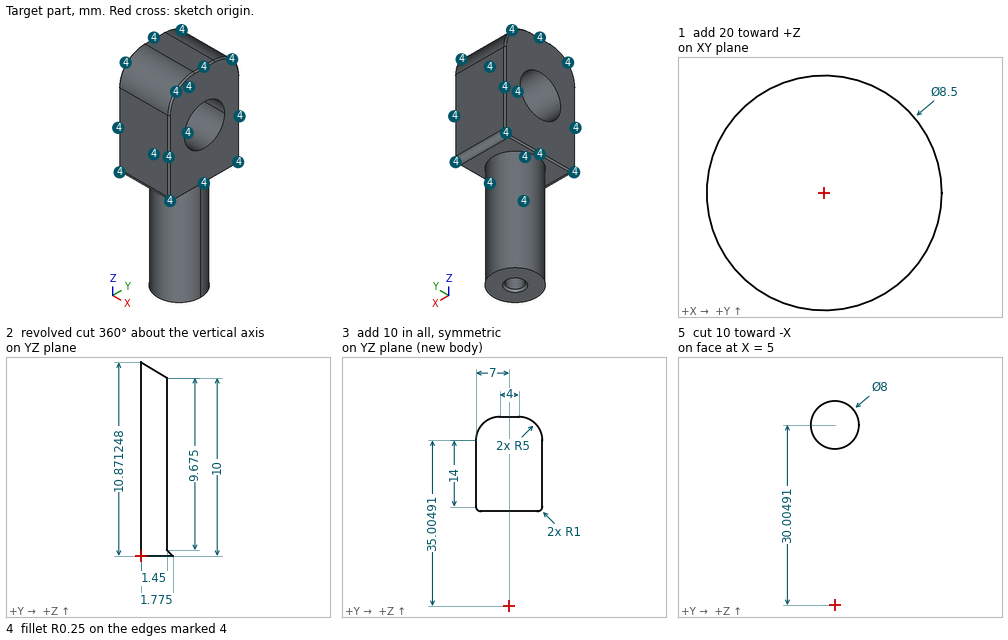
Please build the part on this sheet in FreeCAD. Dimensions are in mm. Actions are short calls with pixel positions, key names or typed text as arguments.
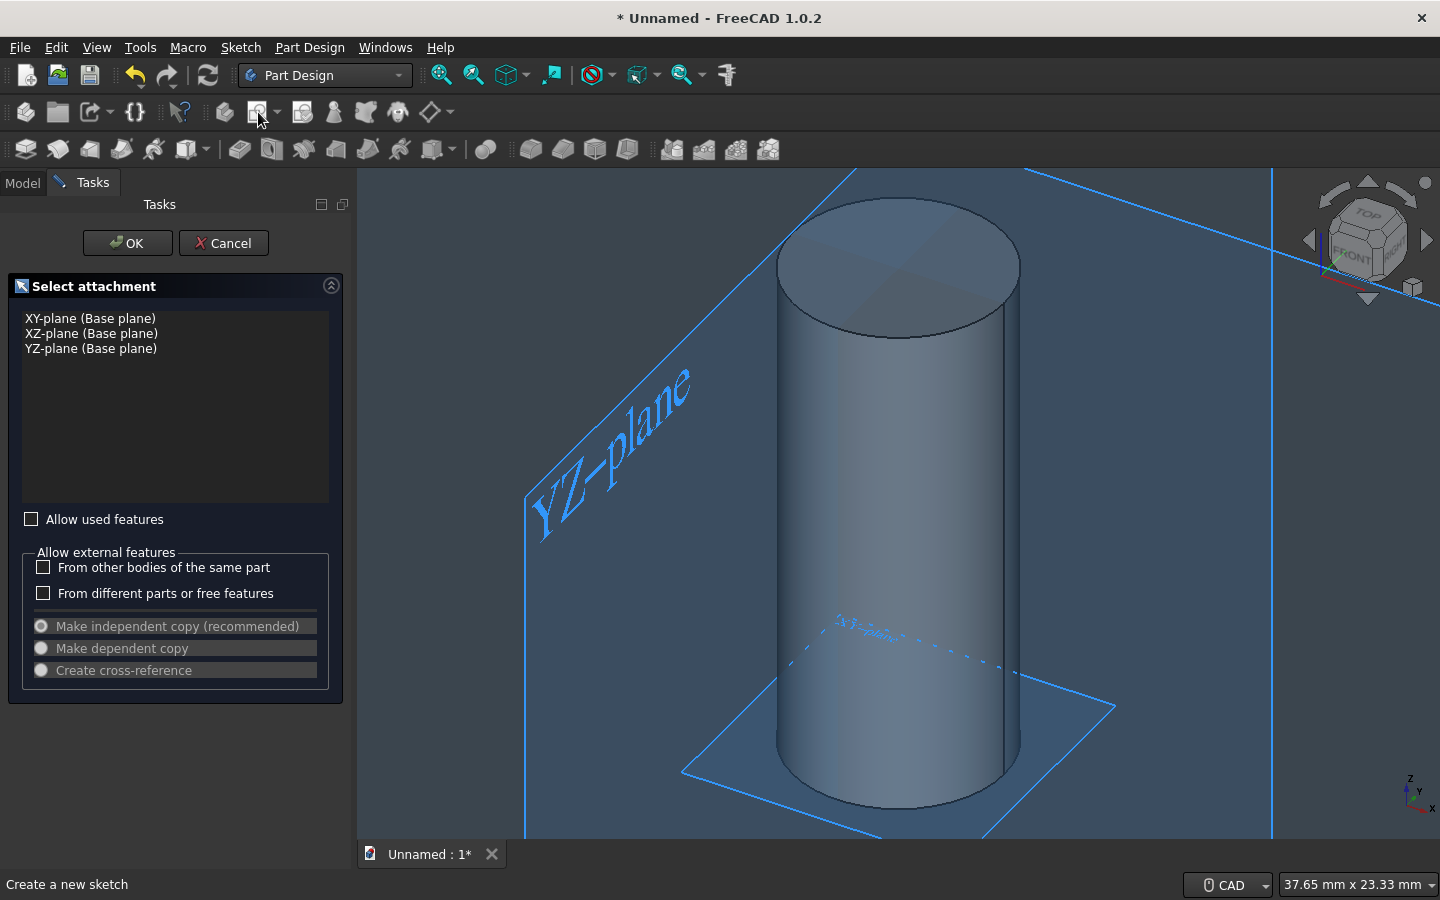
click(82, 348)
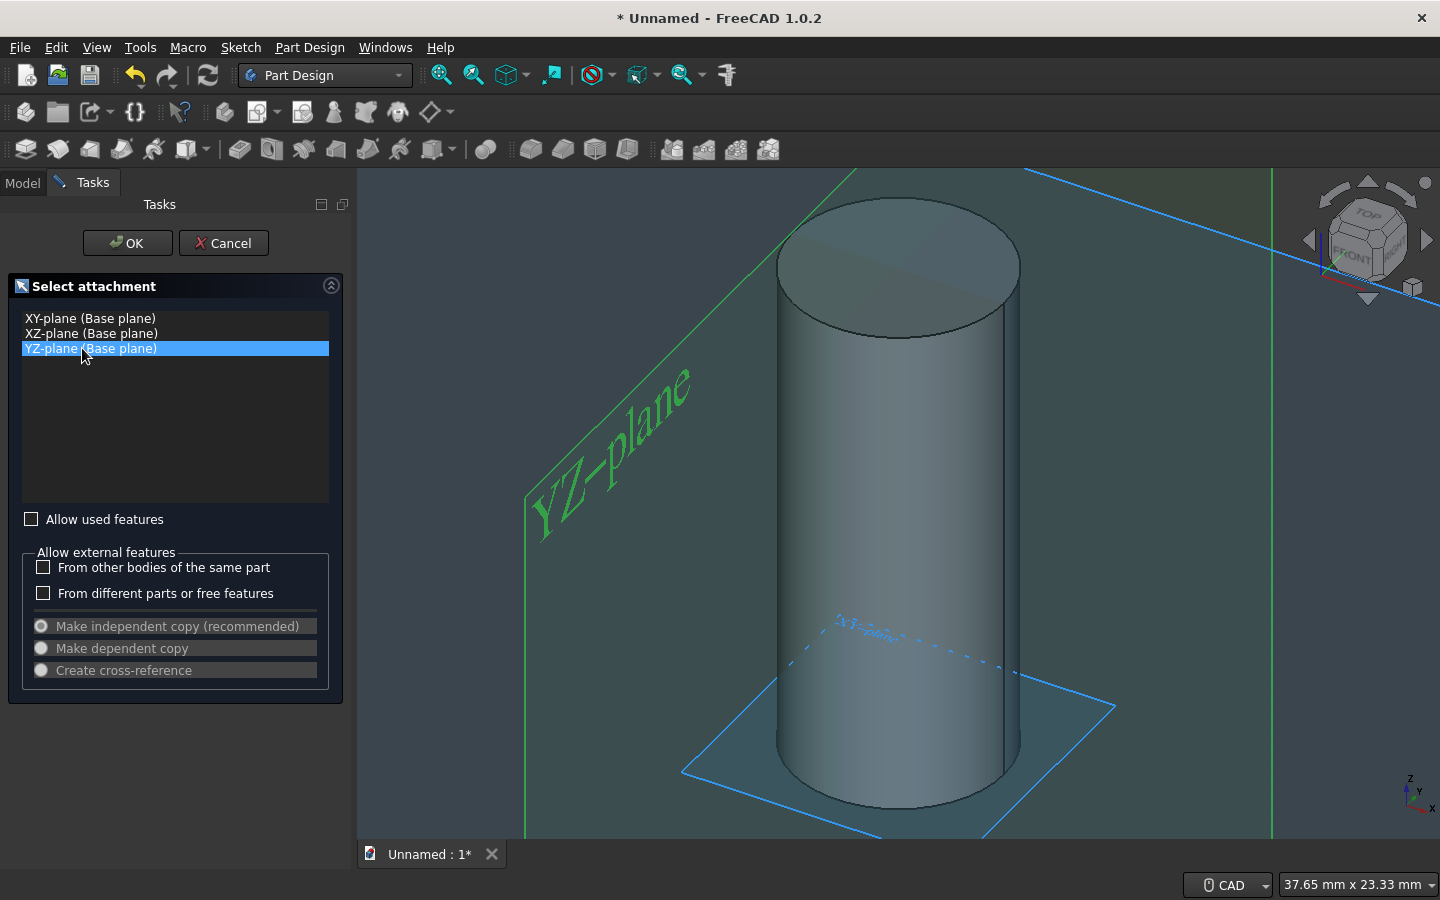
click(128, 243)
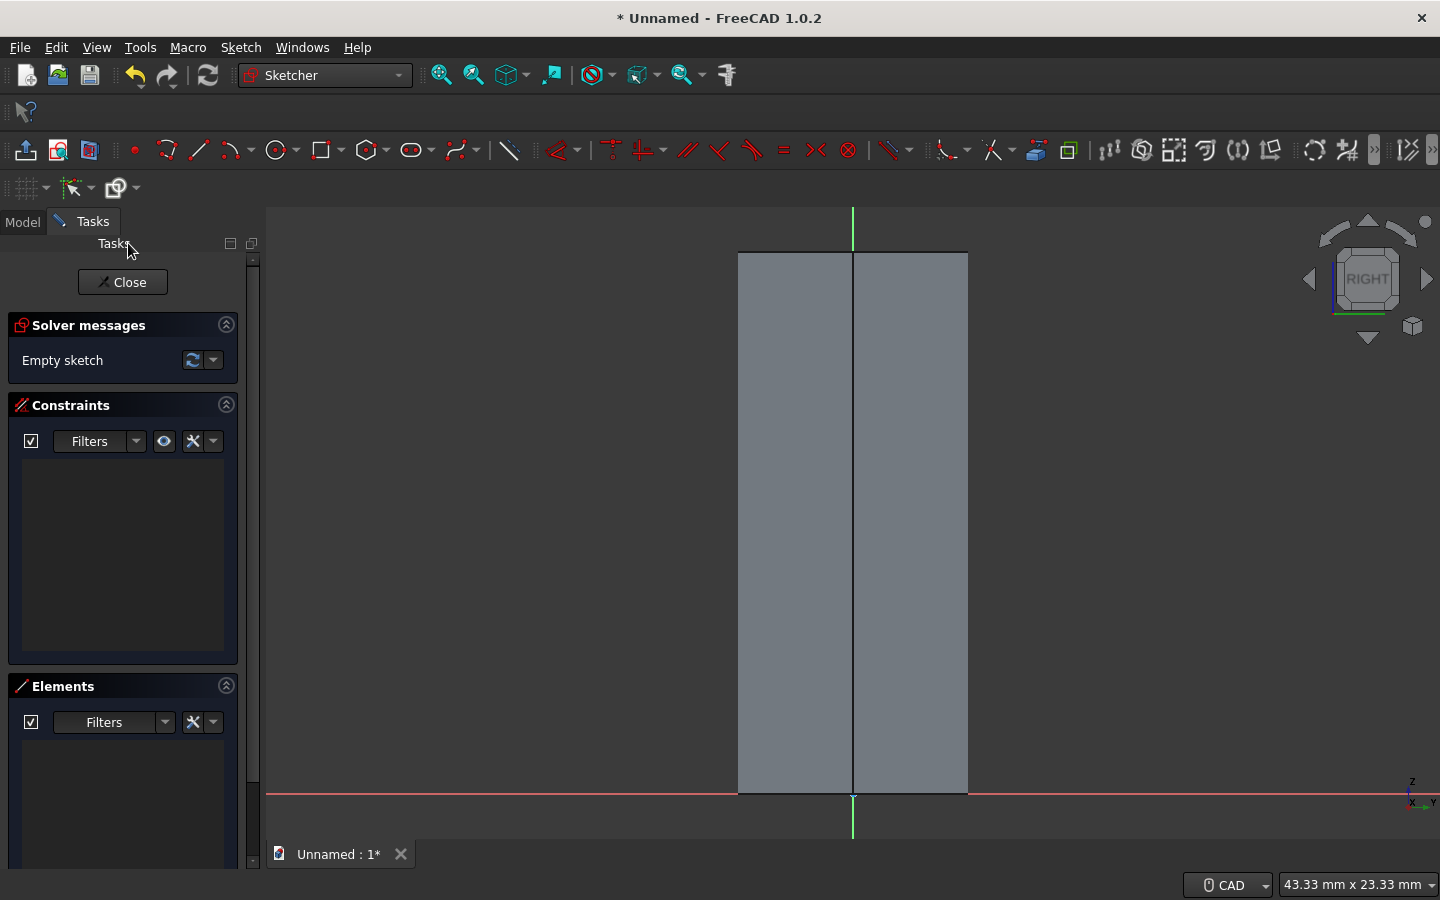
click(90, 150)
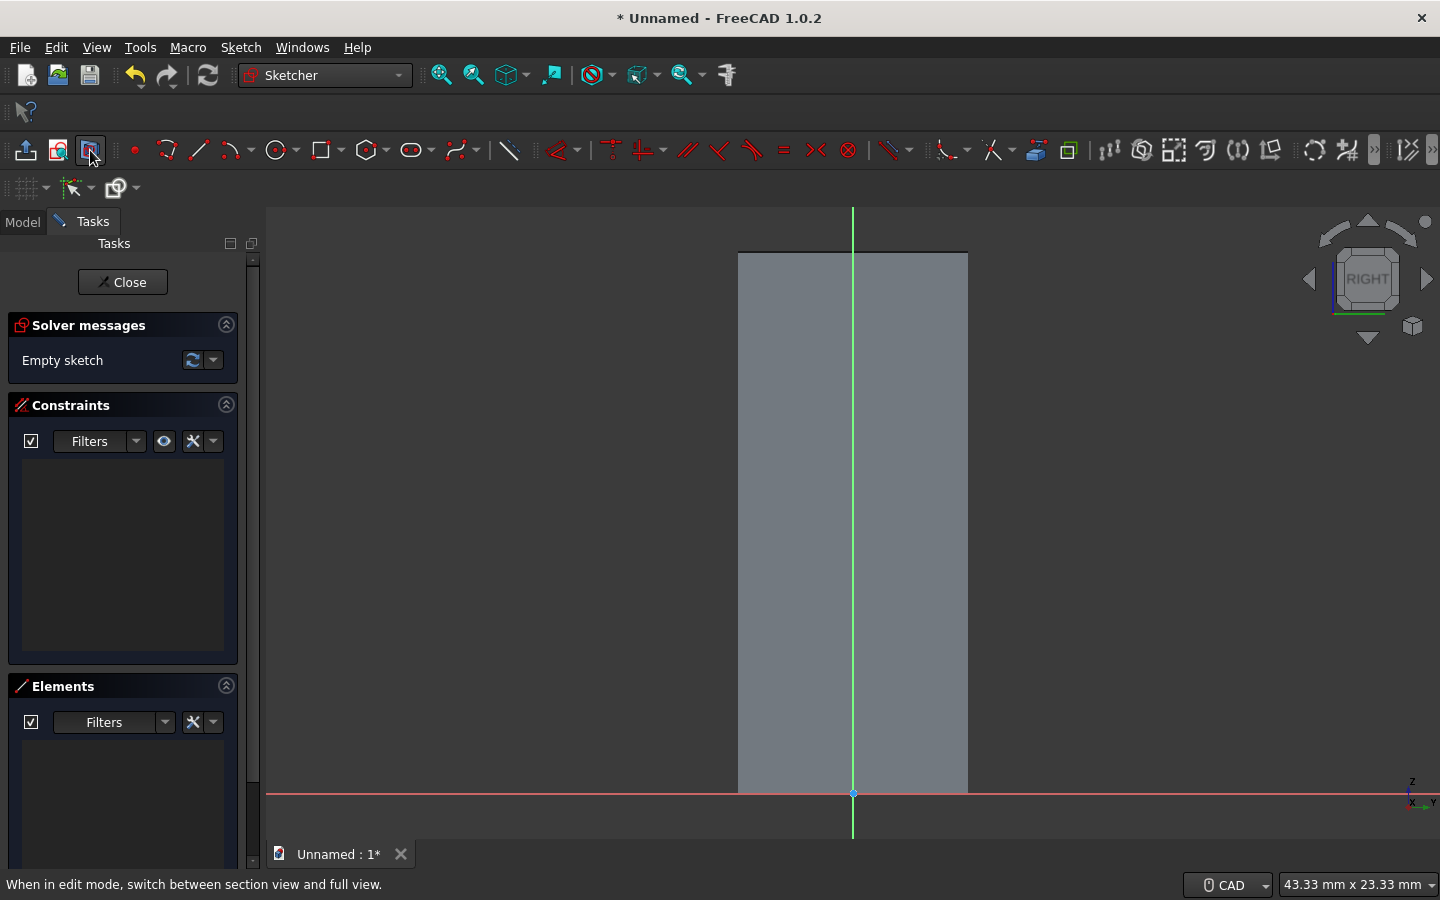
scroll(1065, 811, up, 2)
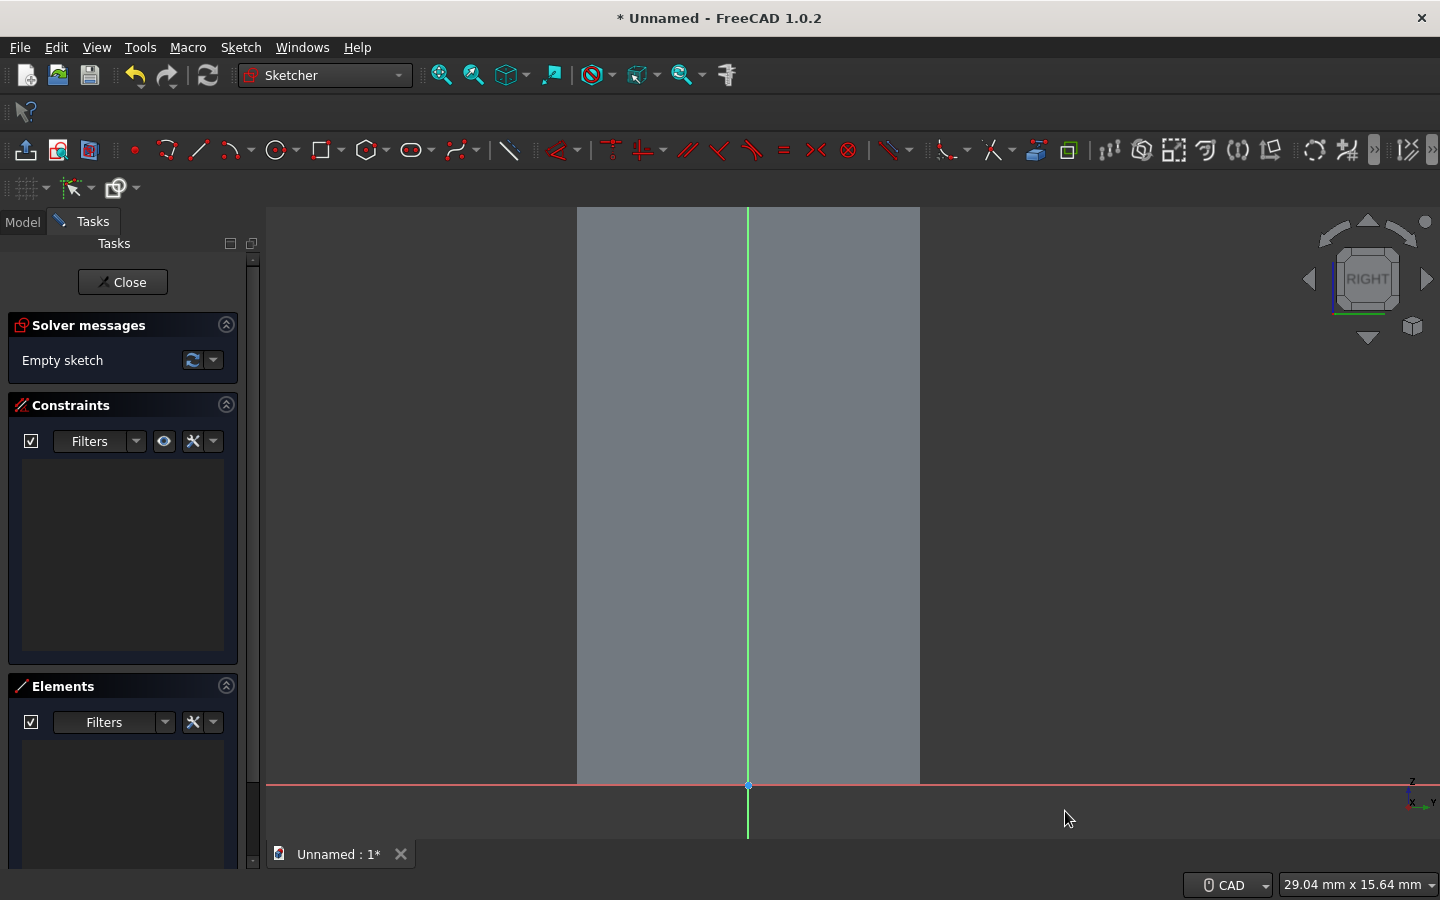
click(168, 150)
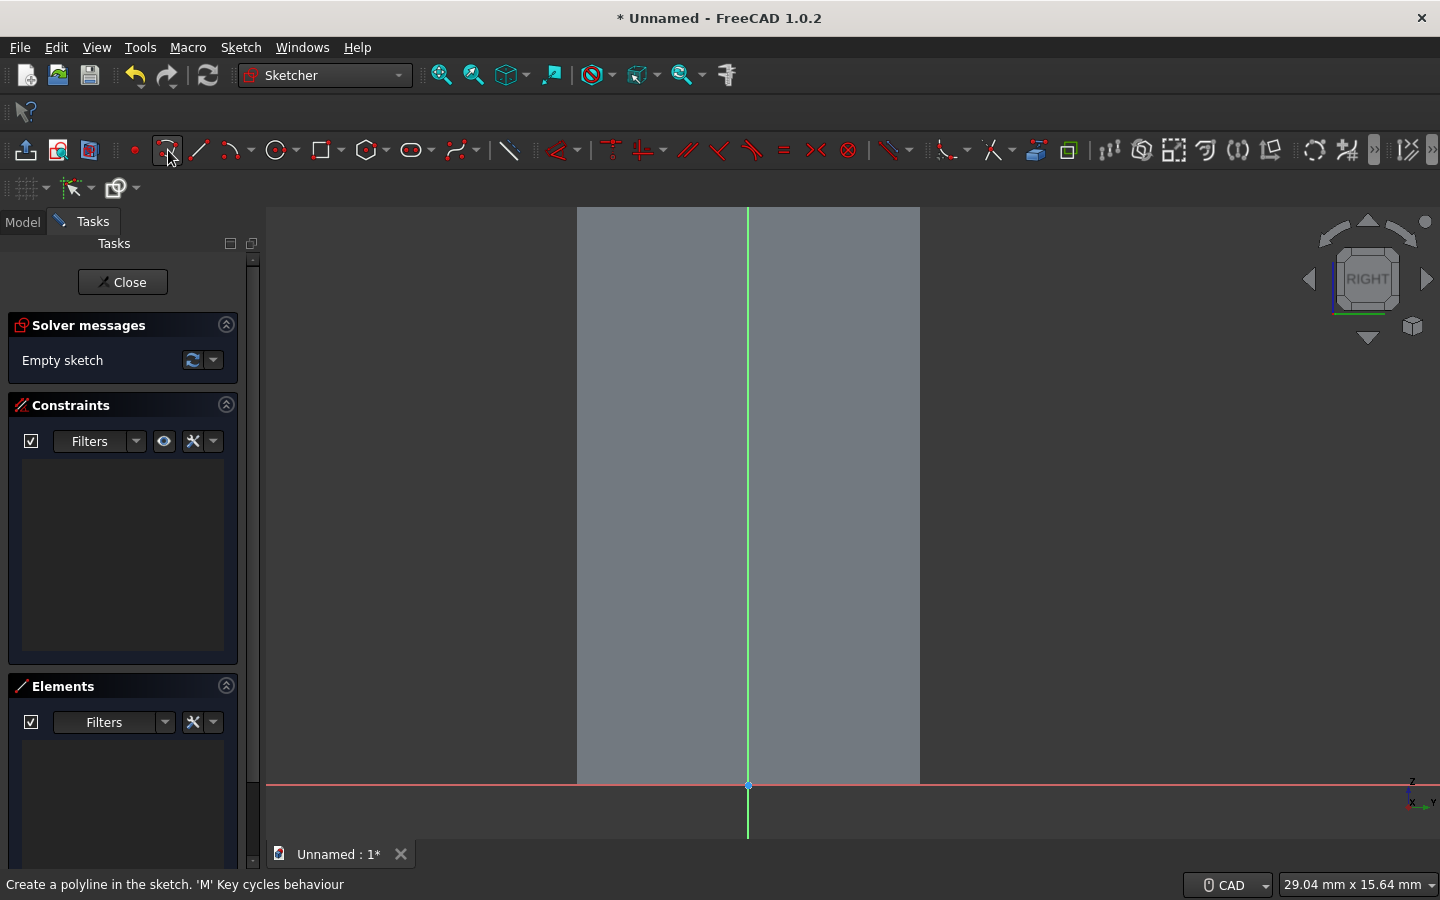
click(748, 785)
click(820, 776)
click(807, 772)
click(807, 381)
click(757, 346)
click(748, 785)
key(Escape)
key(Escape)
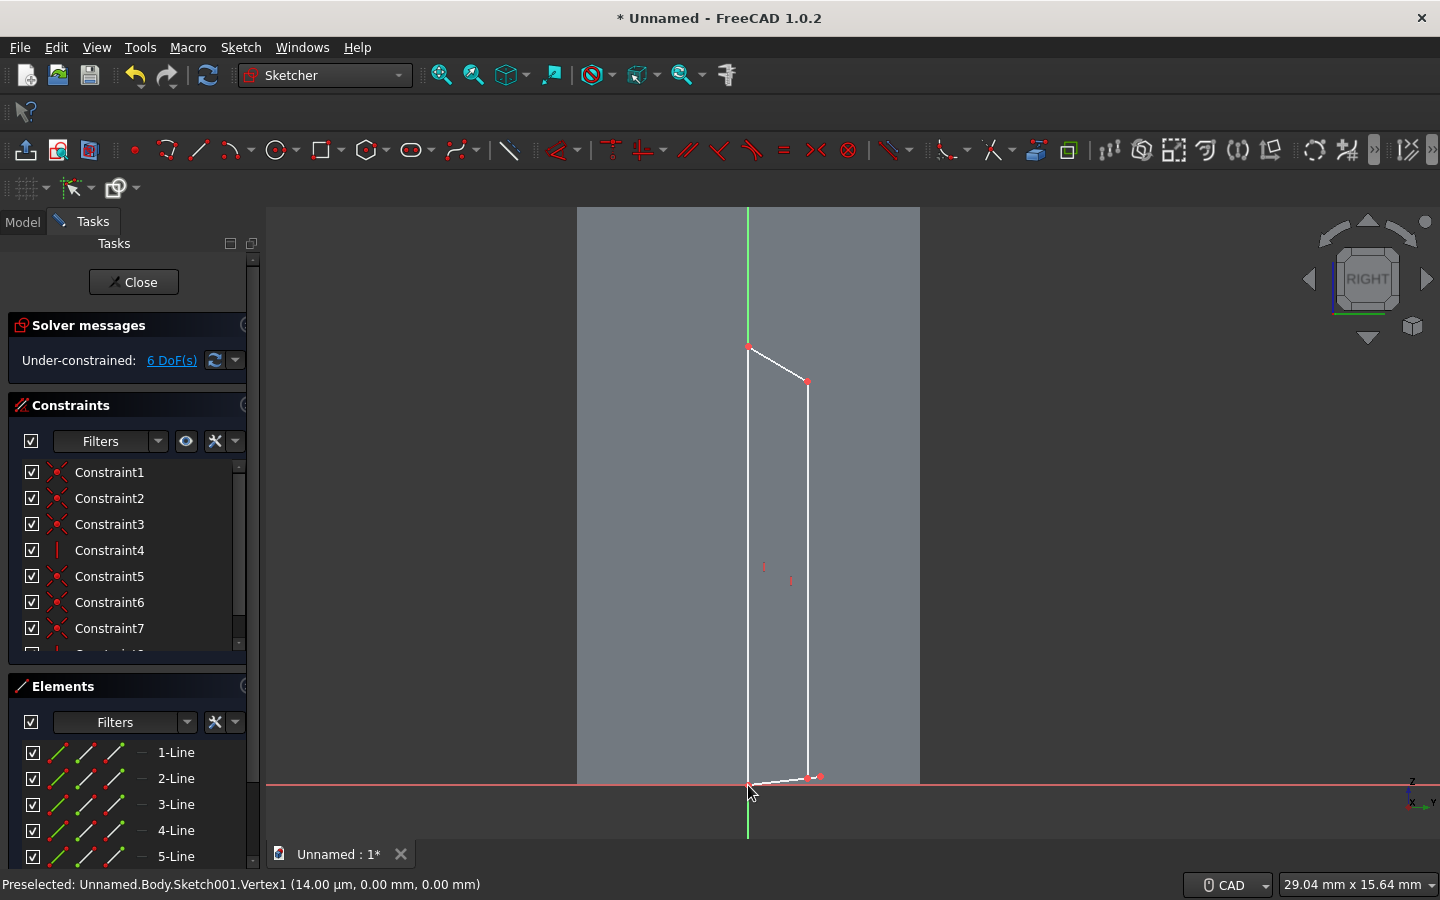
click(770, 783)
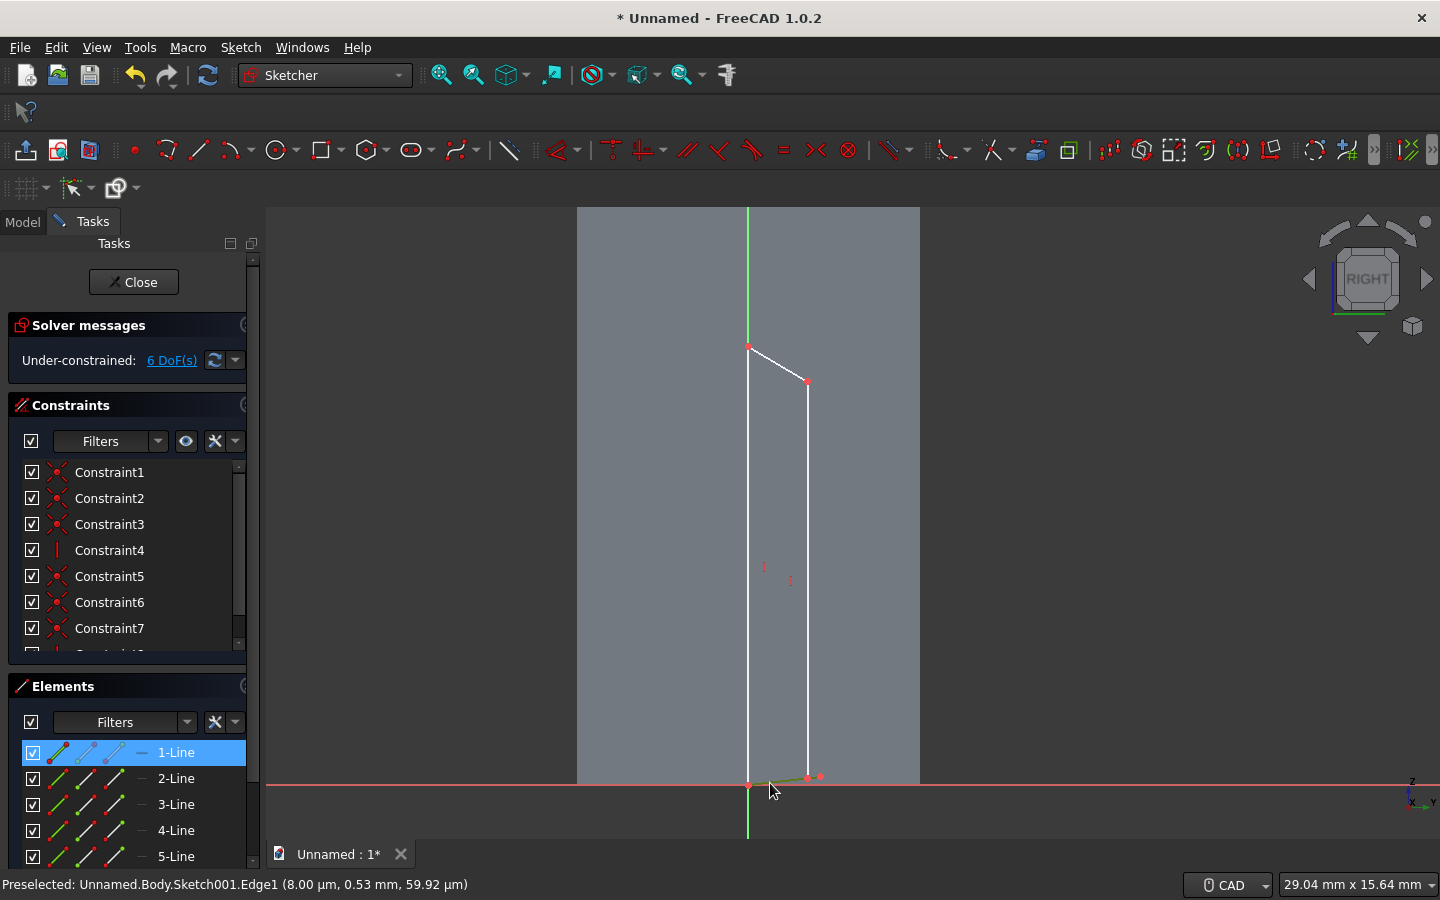
key(h)